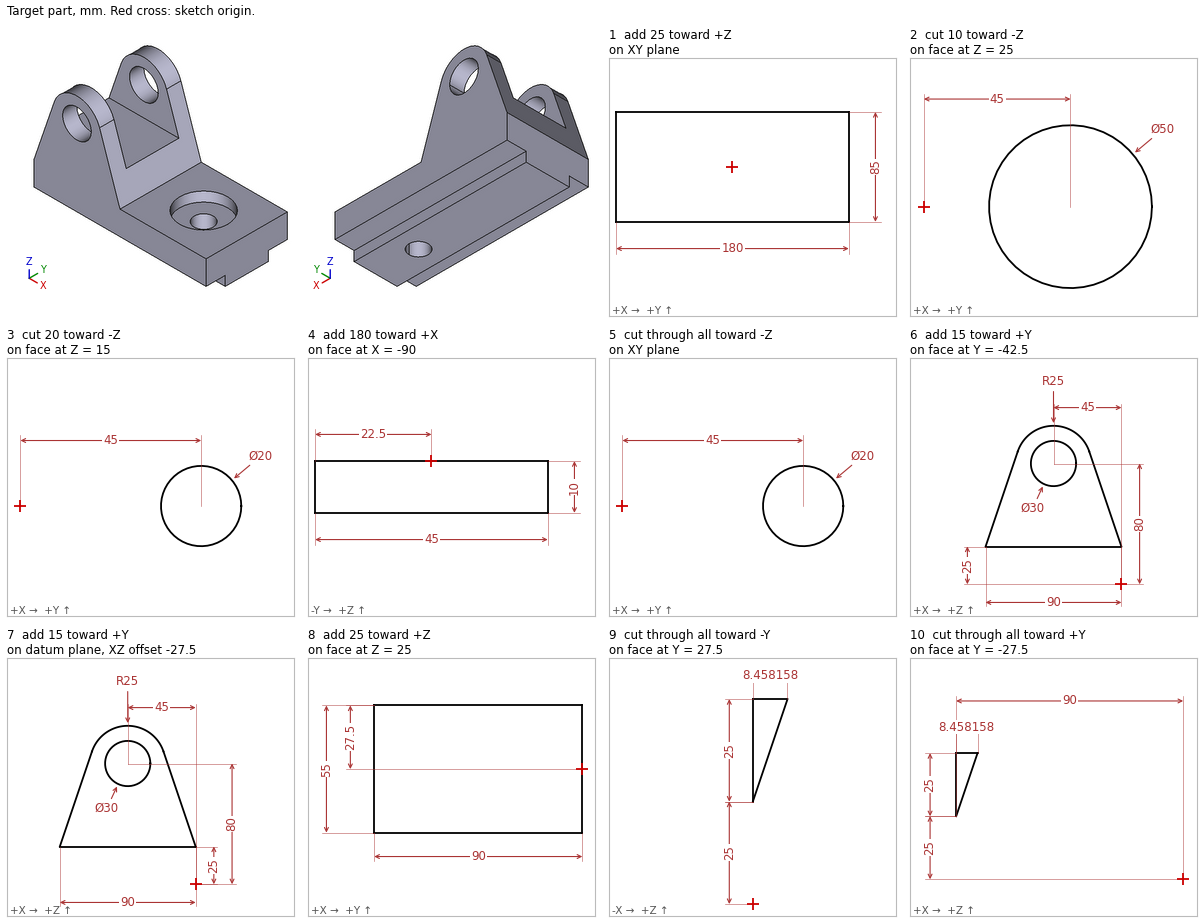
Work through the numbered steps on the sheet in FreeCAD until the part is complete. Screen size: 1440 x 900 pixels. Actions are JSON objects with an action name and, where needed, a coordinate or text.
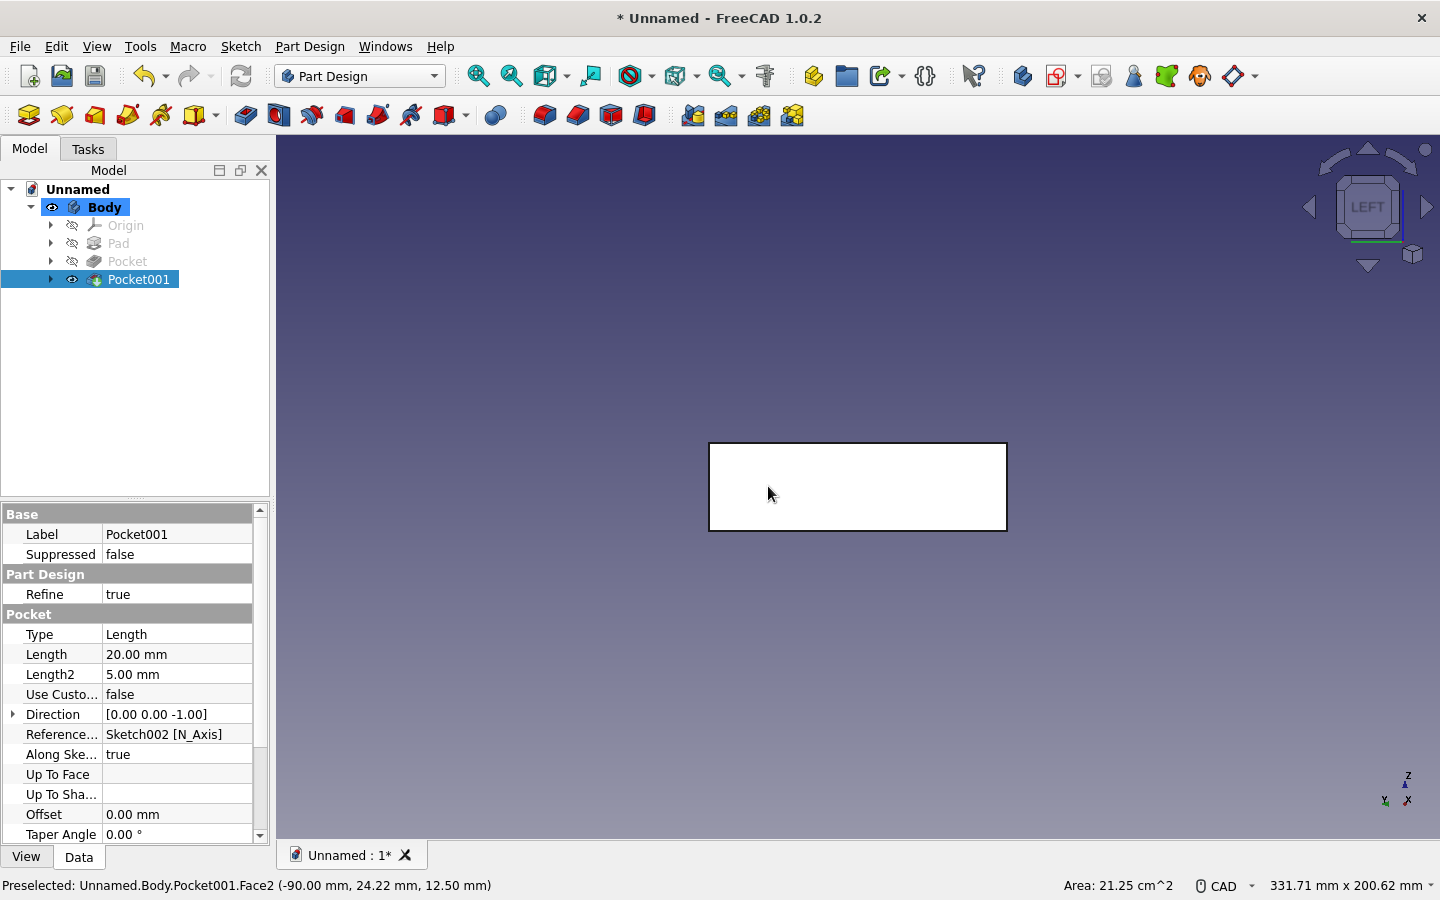
{"action": "left_click", "coordinate": [1056, 76]}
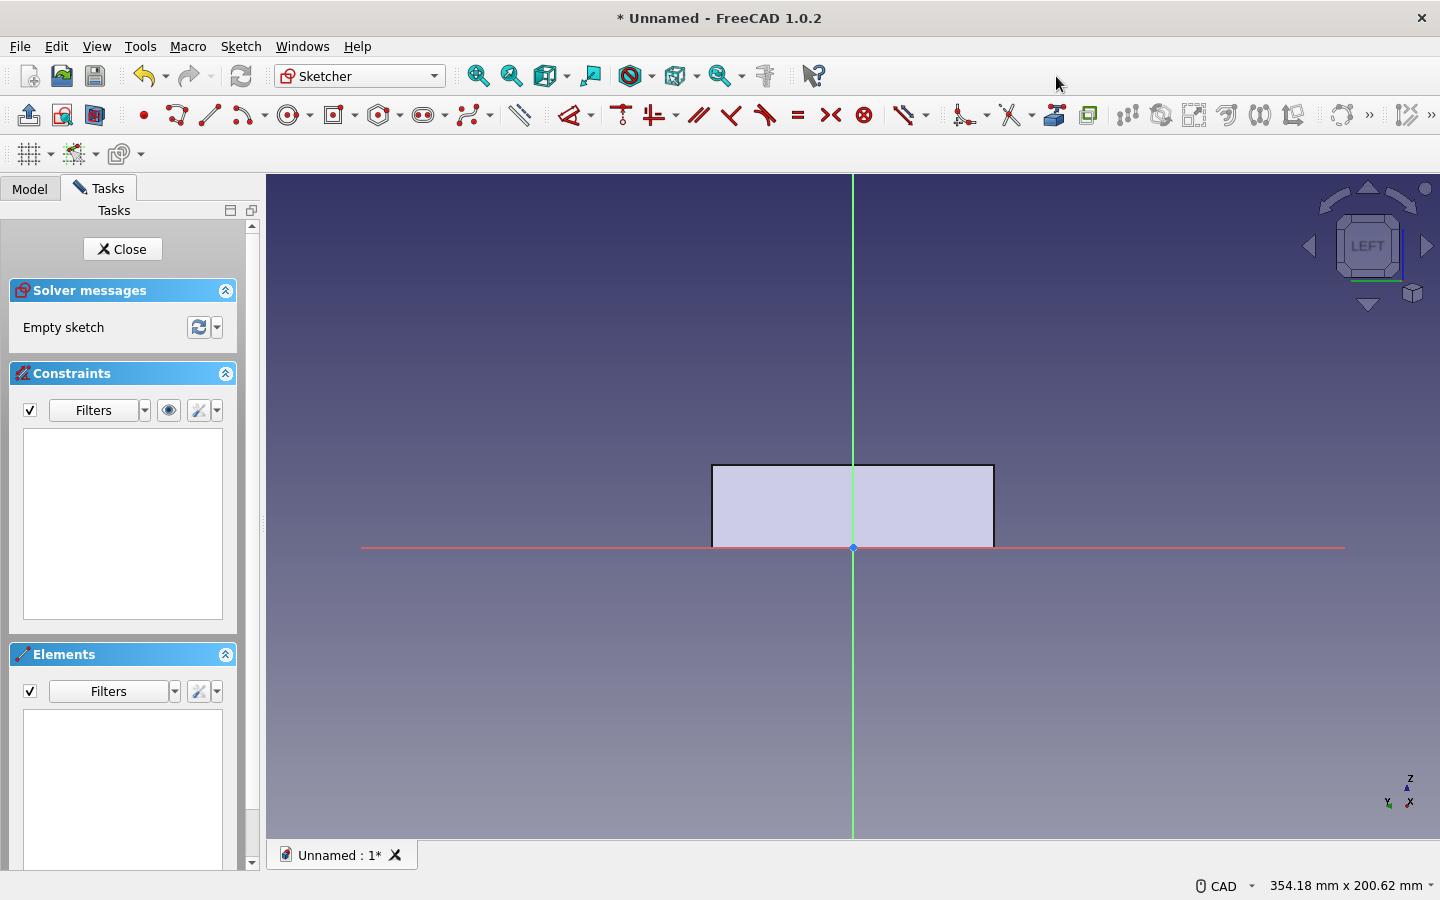
{"action": "scroll", "coordinate": [870, 579], "scroll_direction": "up", "scroll_amount": 8}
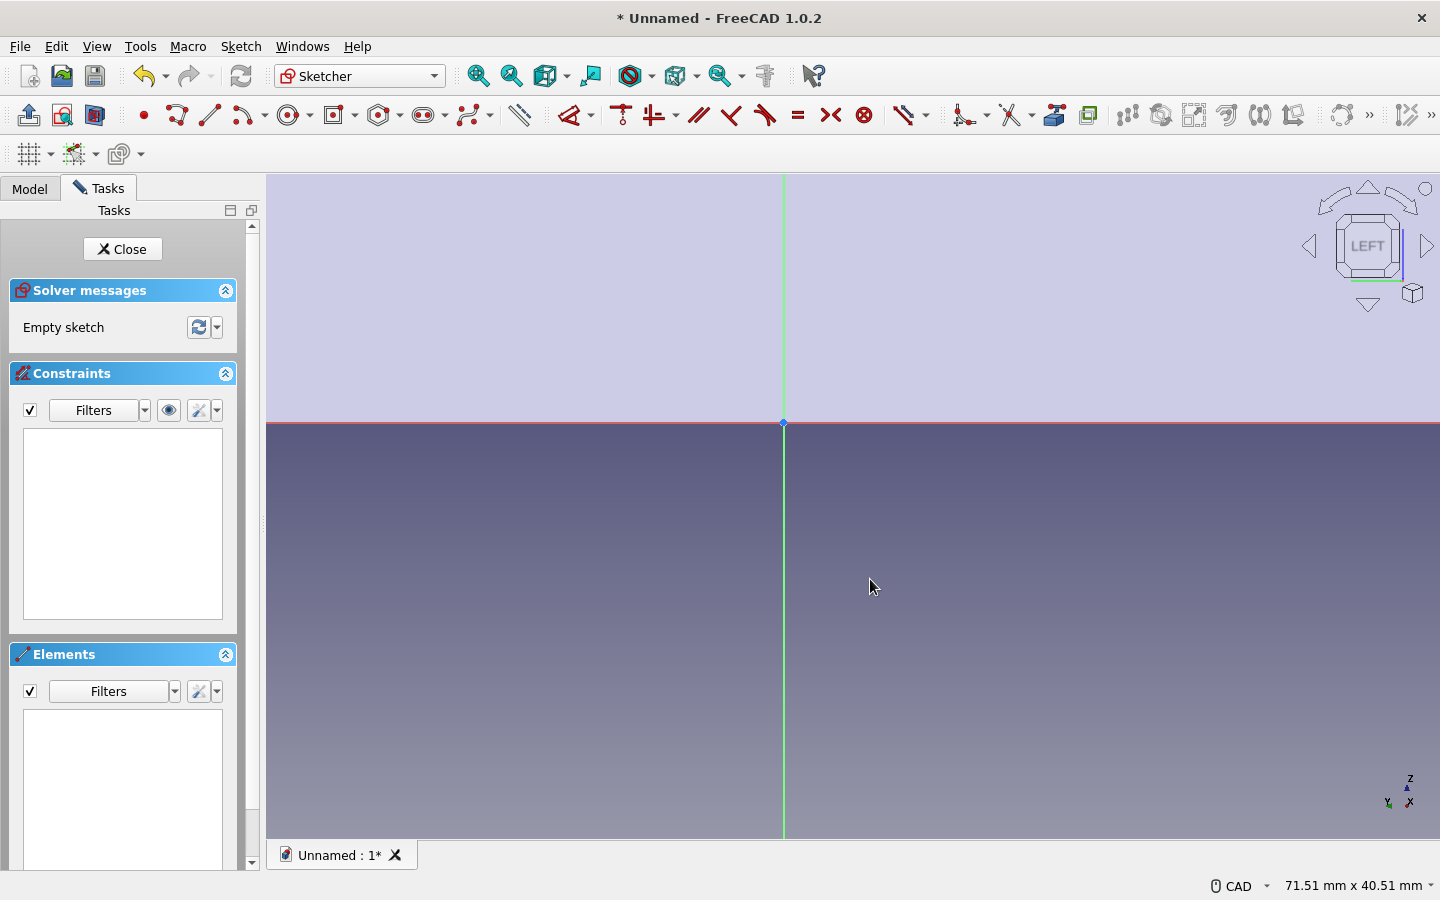
{"action": "key", "text": "g r"}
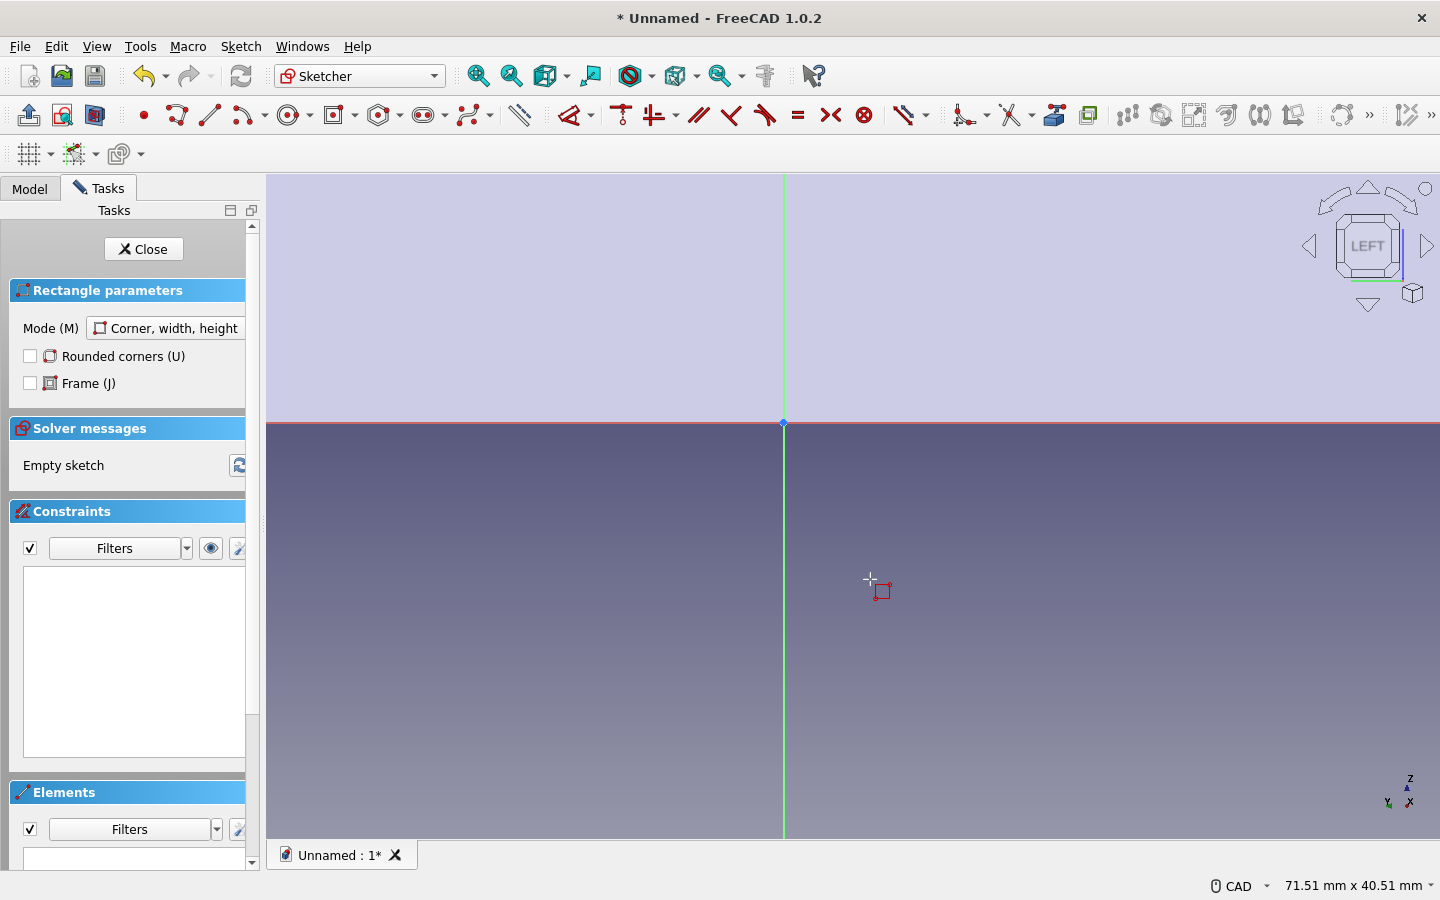
{"action": "left_click", "coordinate": [414, 423]}
{"action": "mouse_move", "coordinate": [1153, 587]}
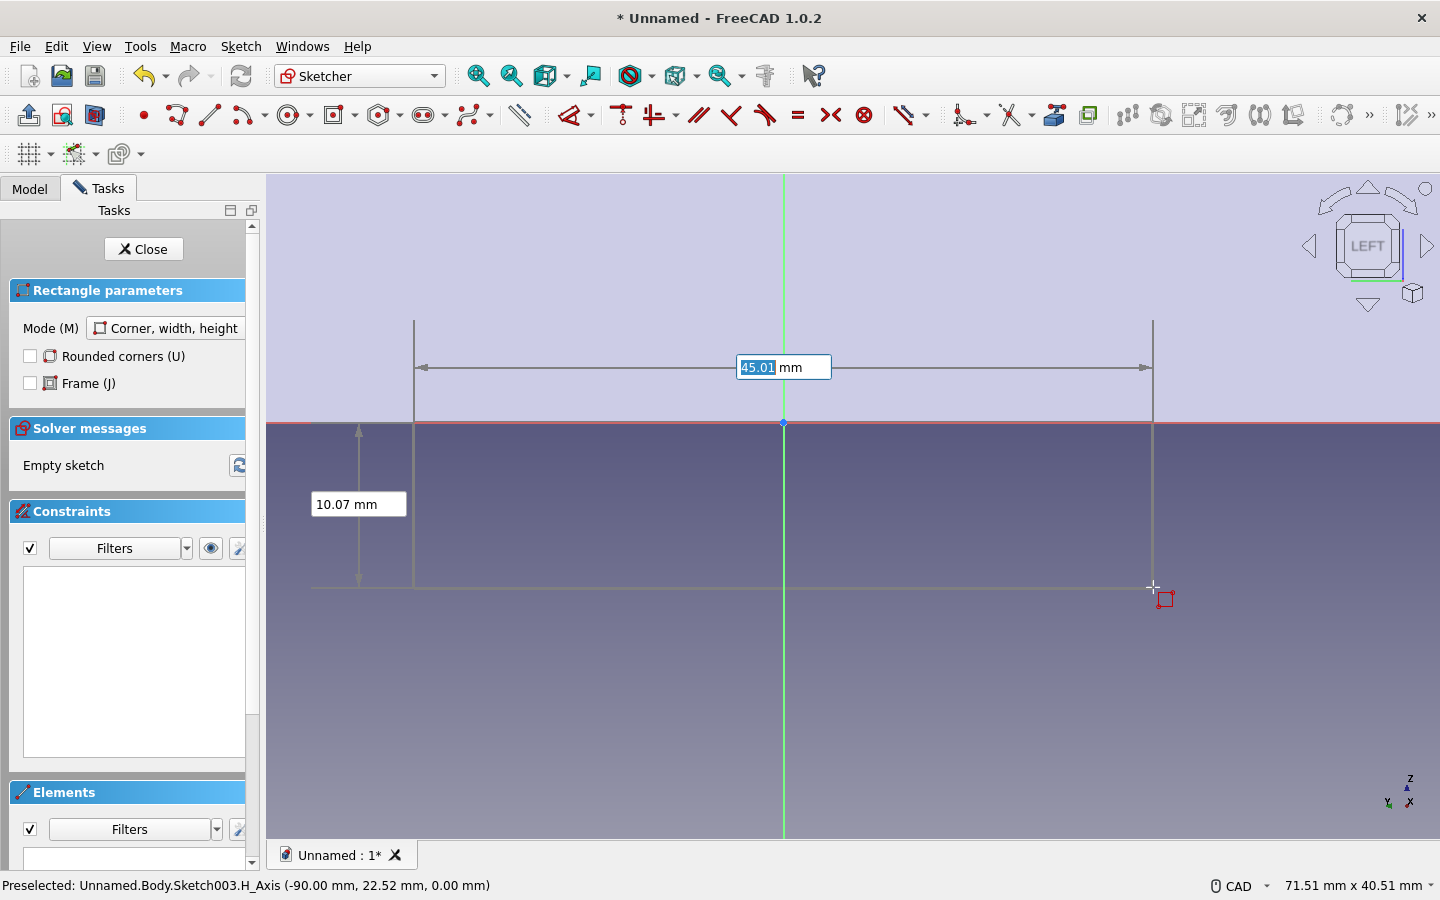
{"action": "type", "text": "45"}
{"action": "key", "text": "Tab"}
{"action": "type", "text": "10"}
{"action": "key", "text": "Return"}
{"action": "key", "text": "Escape"}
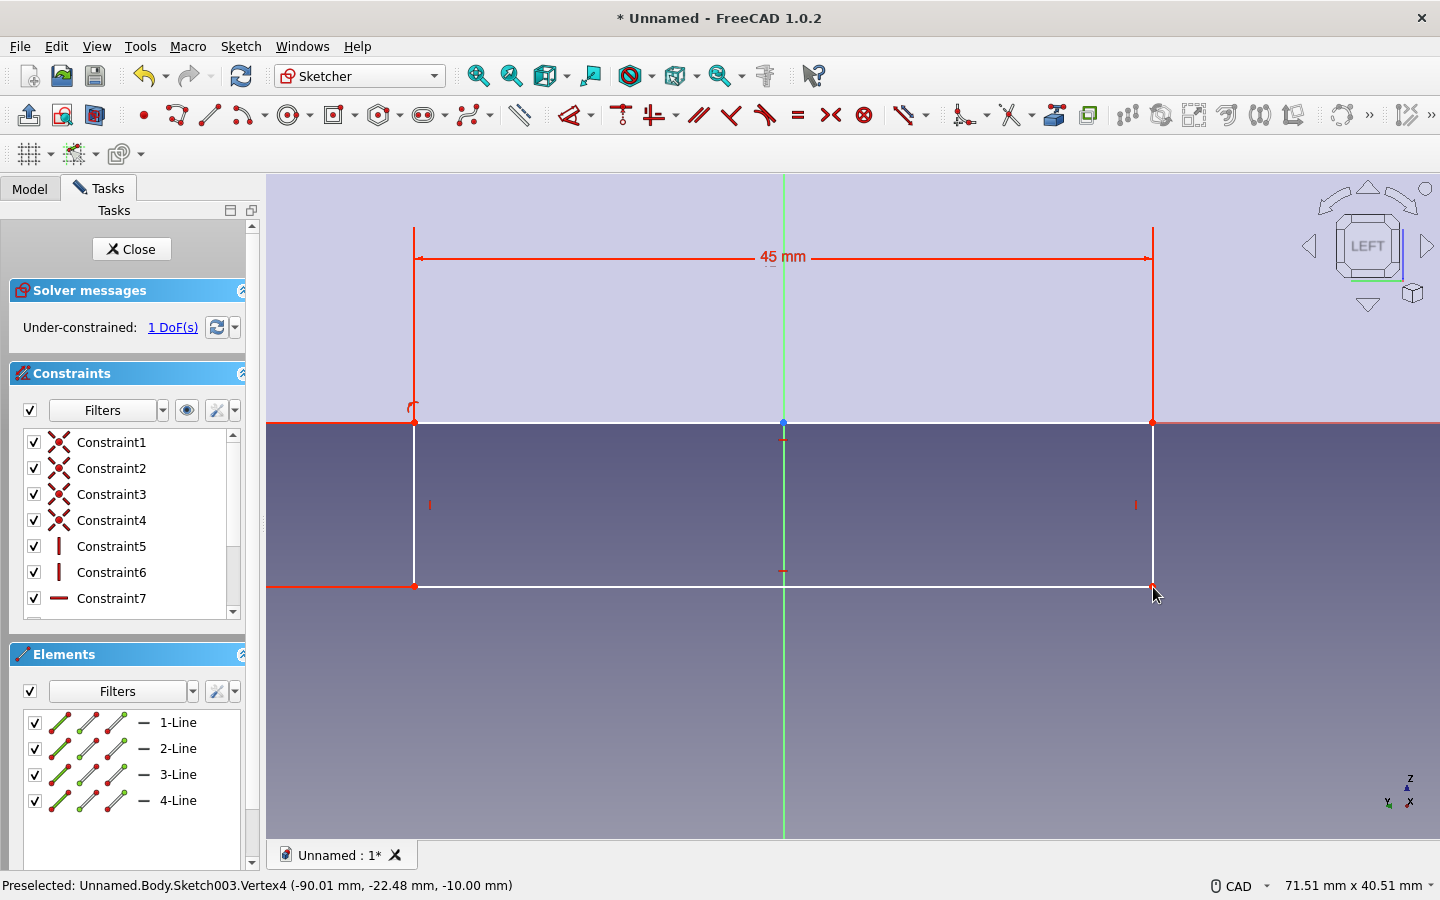
{"action": "left_click", "coordinate": [568, 116]}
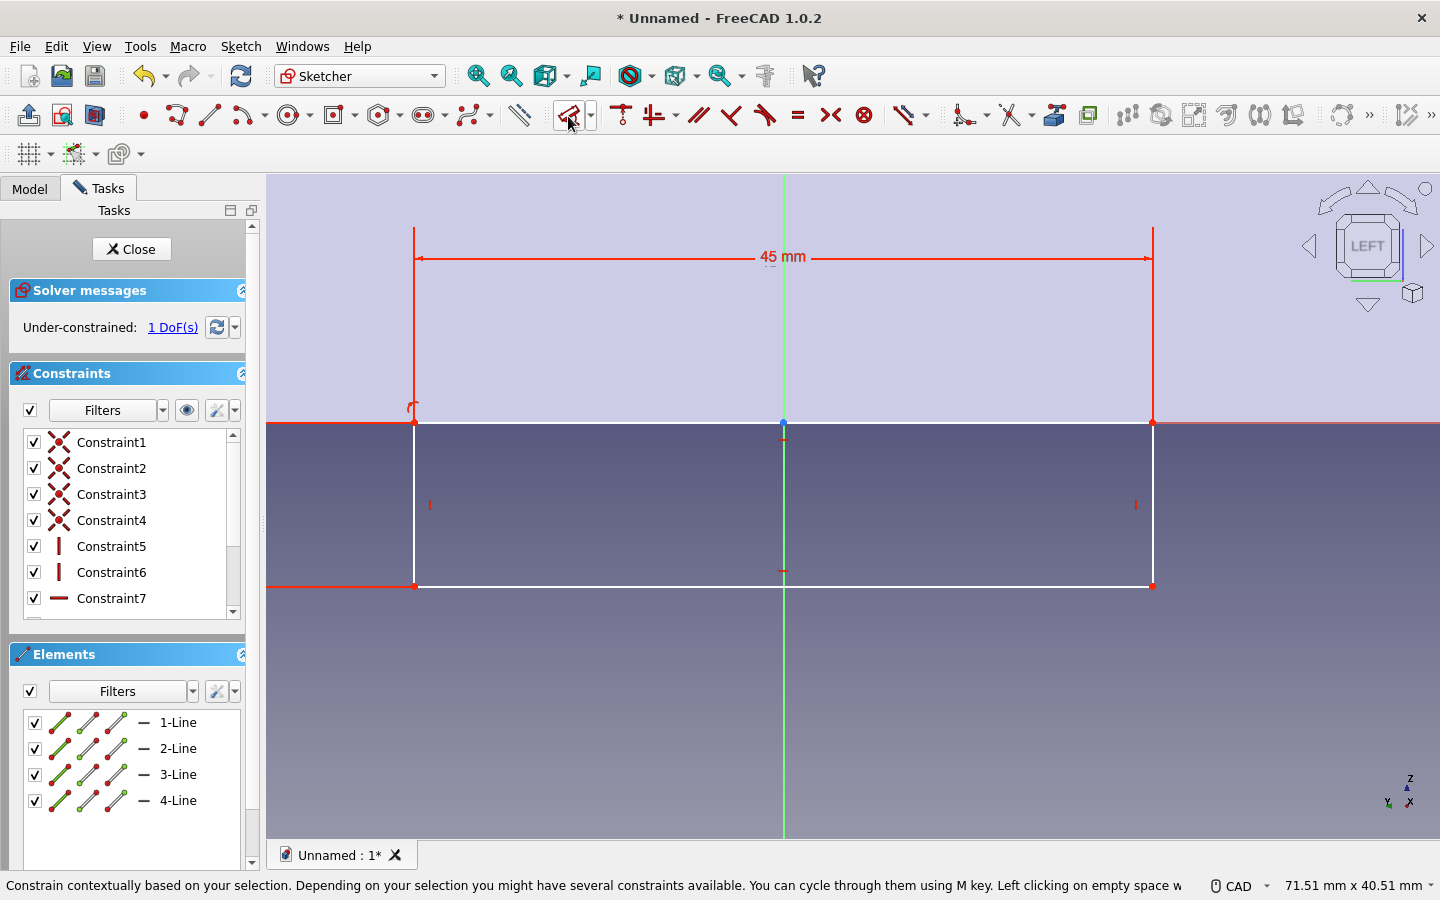
{"action": "left_click", "coordinate": [414, 423]}
{"action": "left_click", "coordinate": [599, 389]}